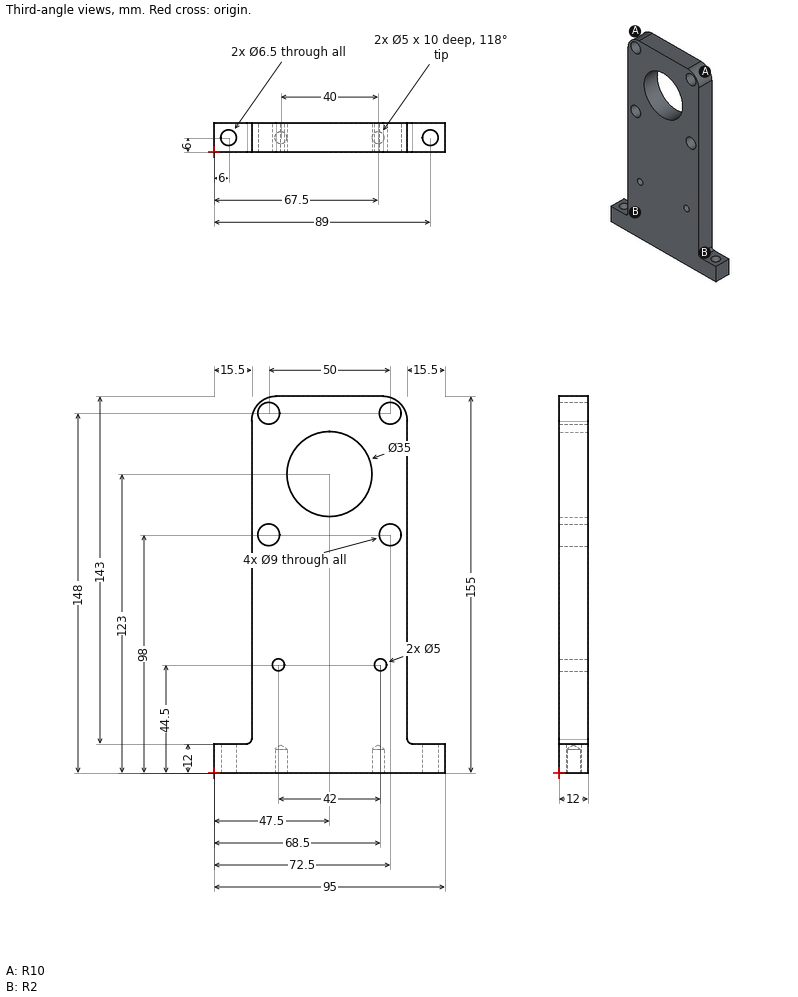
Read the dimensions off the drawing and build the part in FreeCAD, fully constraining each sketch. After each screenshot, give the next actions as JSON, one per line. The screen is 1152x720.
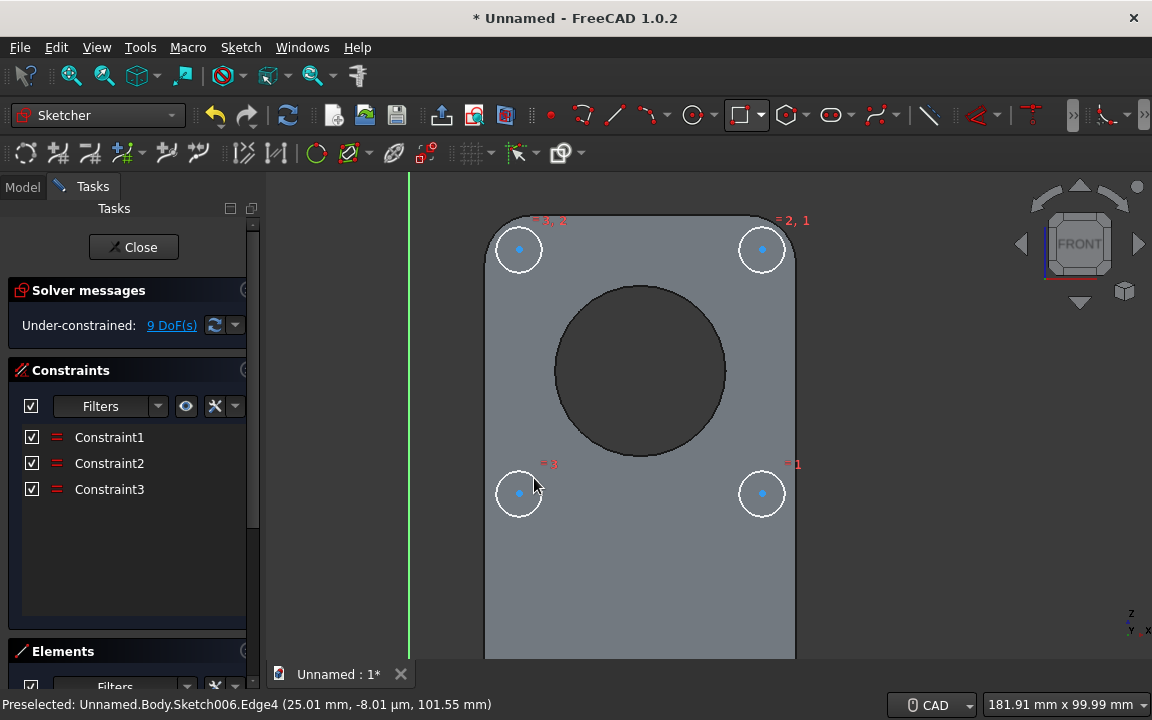
{"action": "left_click", "coordinate": [762, 494]}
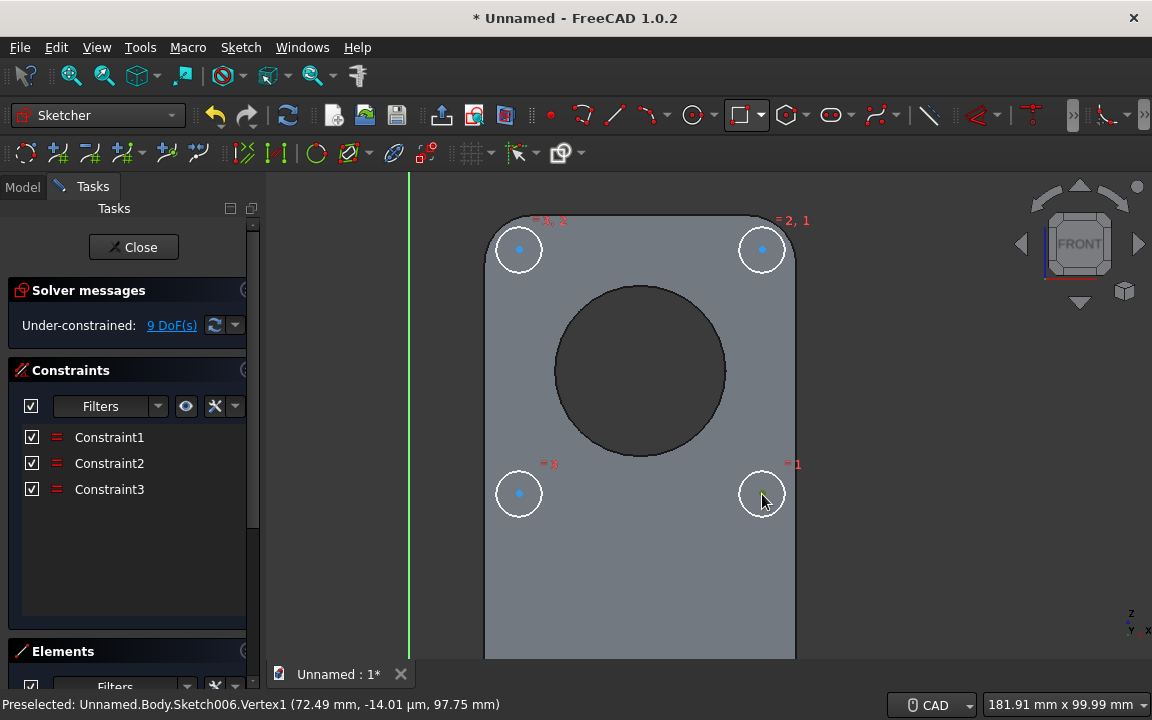
{"action": "left_click", "coordinate": [762, 250]}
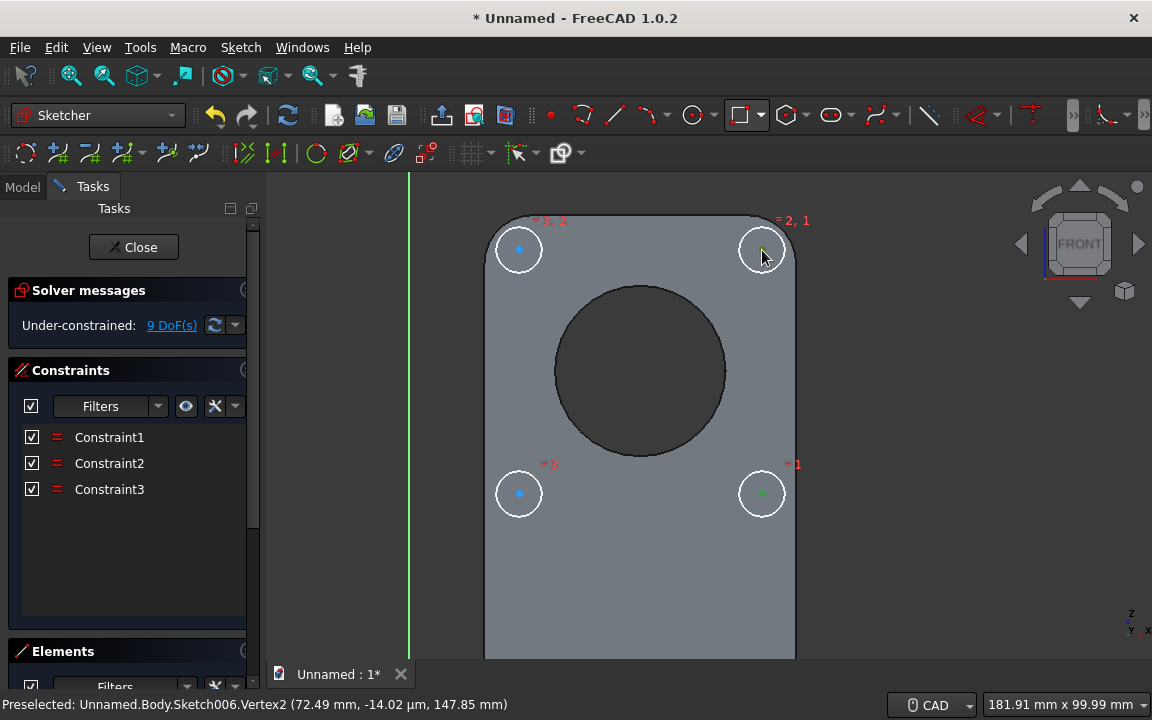
{"action": "key", "text": "v"}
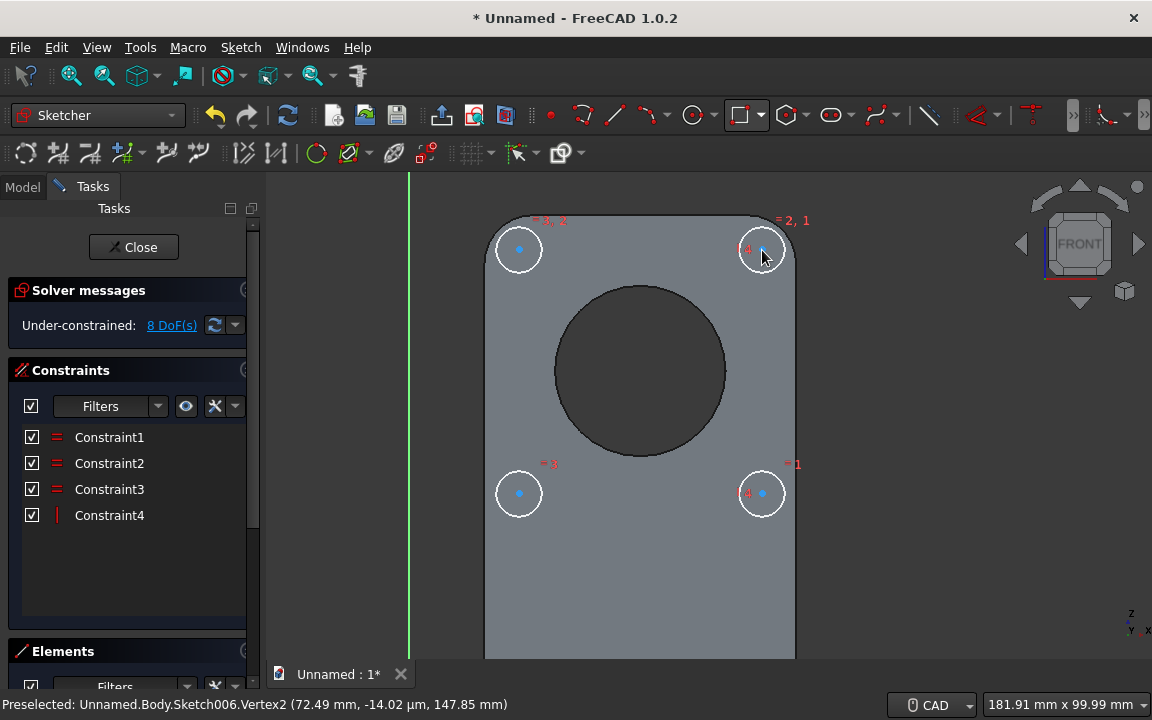
{"action": "left_click", "coordinate": [762, 250]}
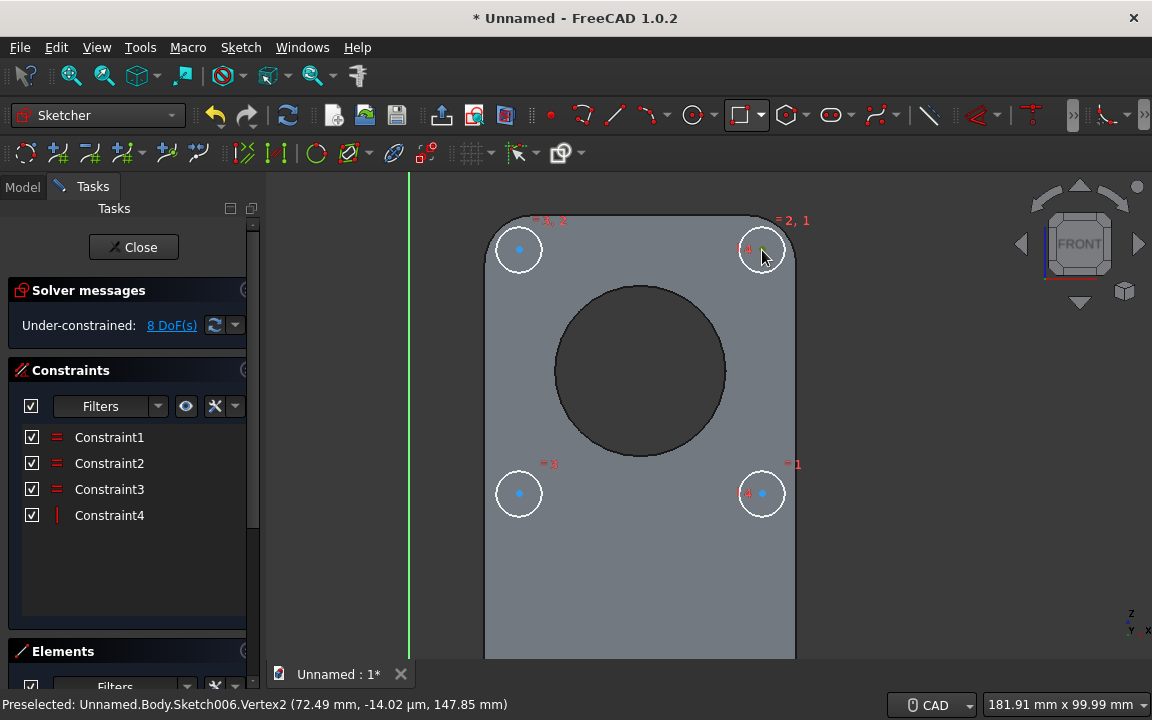
{"action": "left_click", "coordinate": [519, 250]}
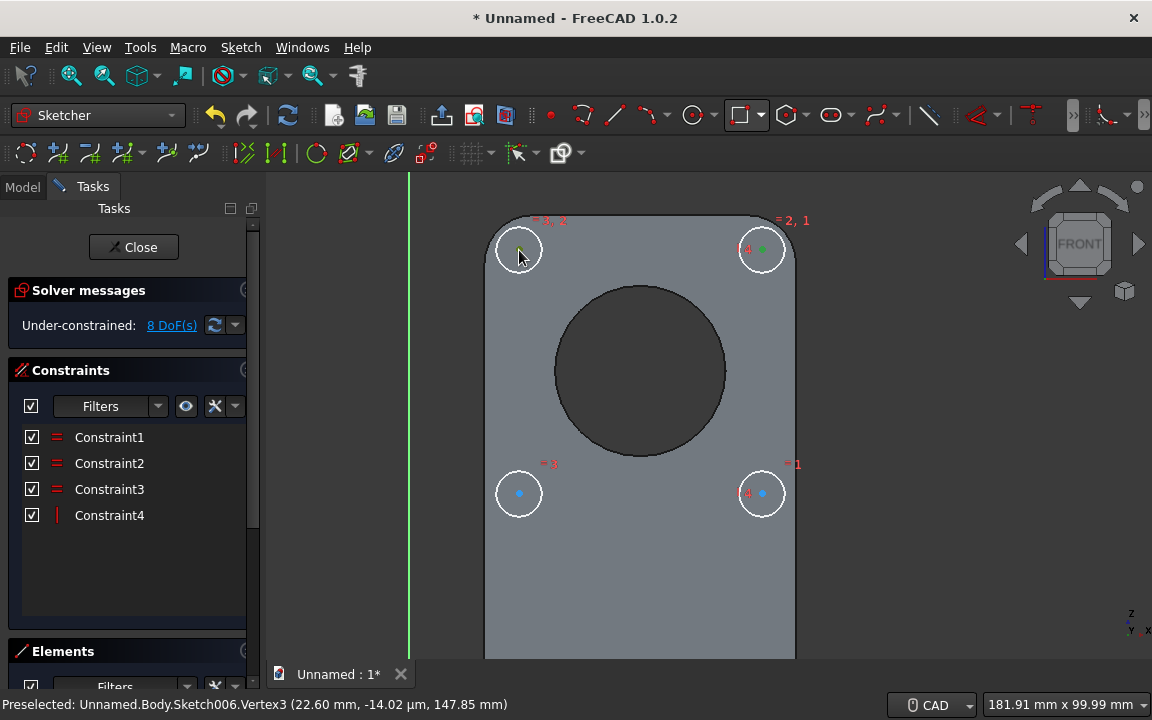
{"action": "key", "text": "h"}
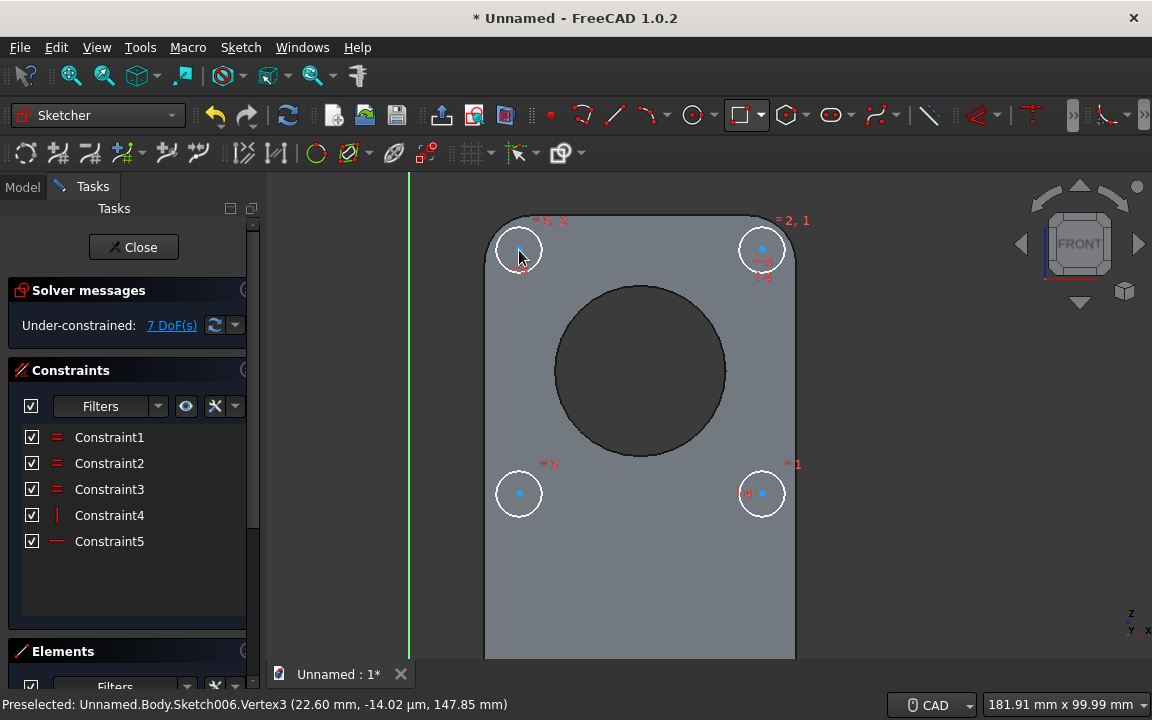
{"action": "left_click", "coordinate": [519, 250]}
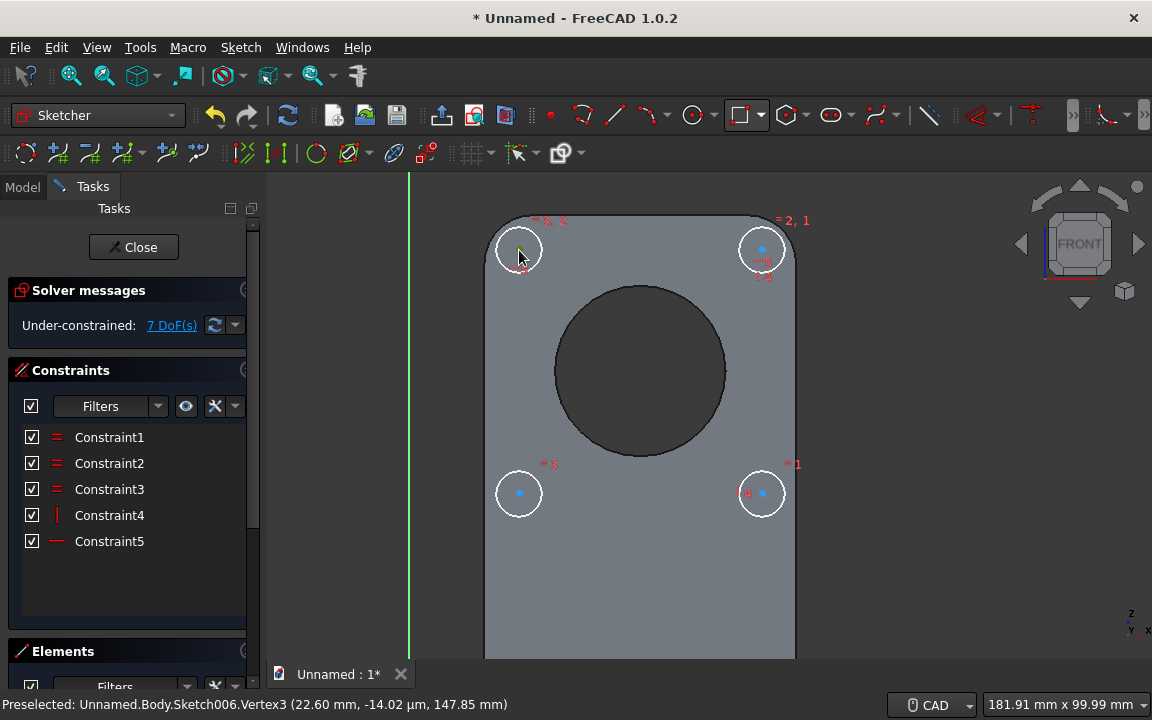
{"action": "left_click", "coordinate": [519, 494]}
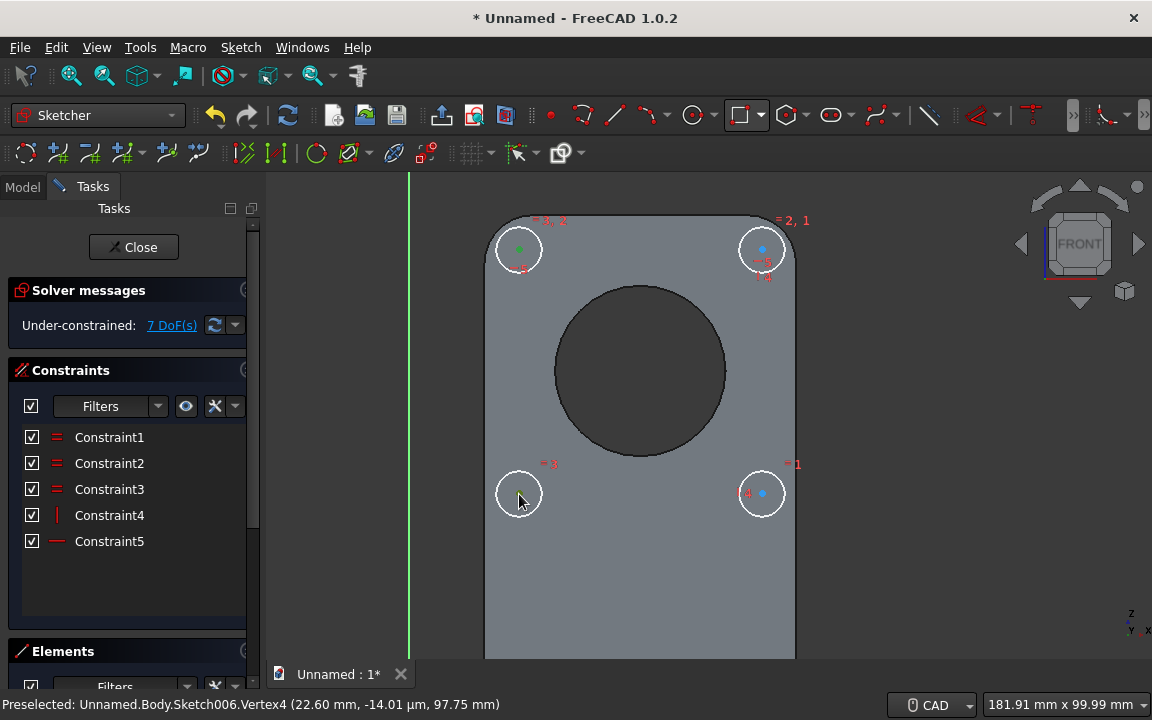
{"action": "key", "text": "v"}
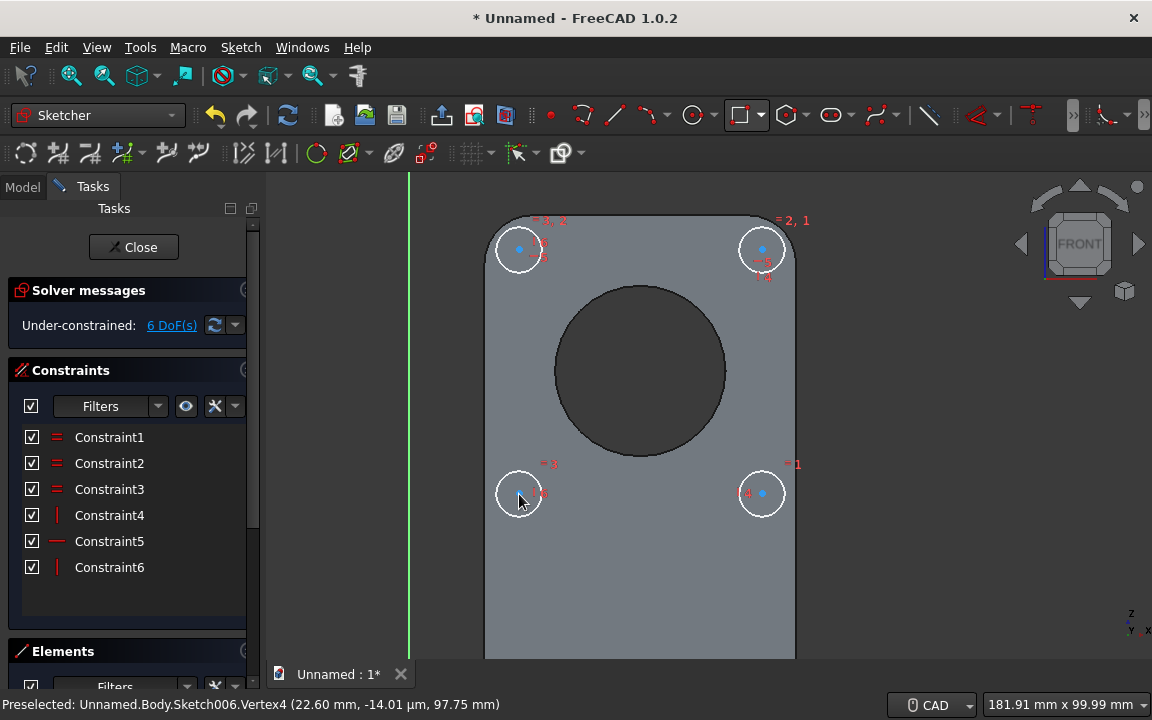
{"action": "left_click", "coordinate": [762, 494]}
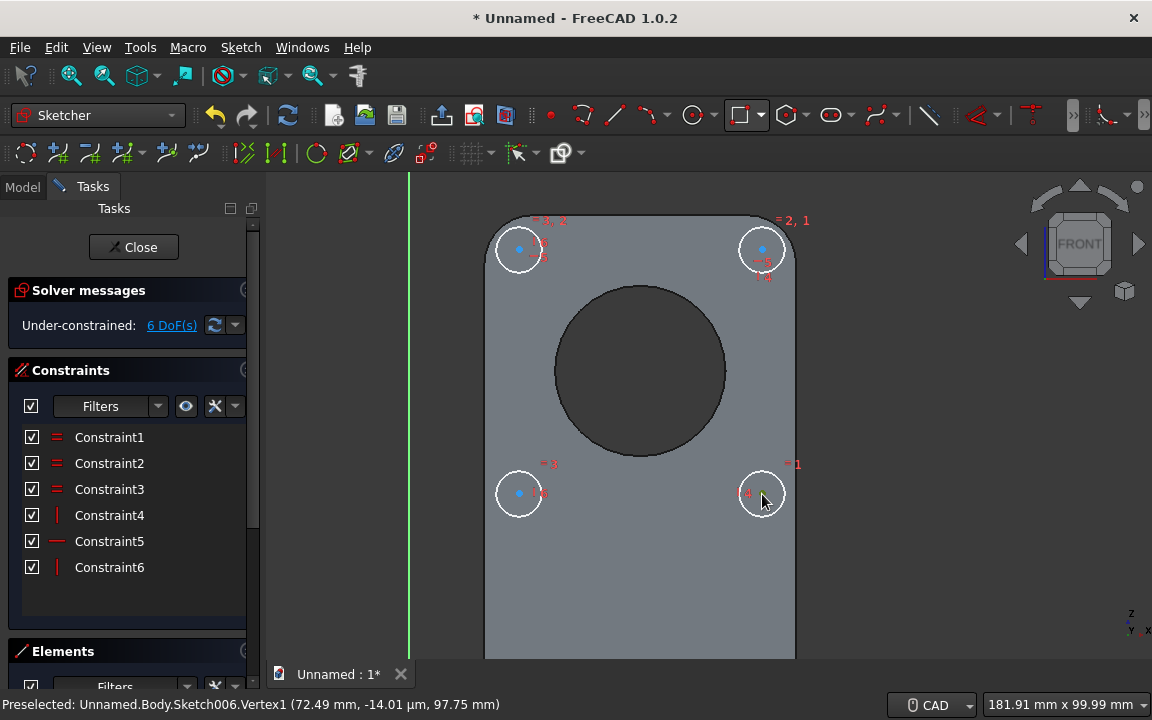
{"action": "left_click", "coordinate": [519, 494]}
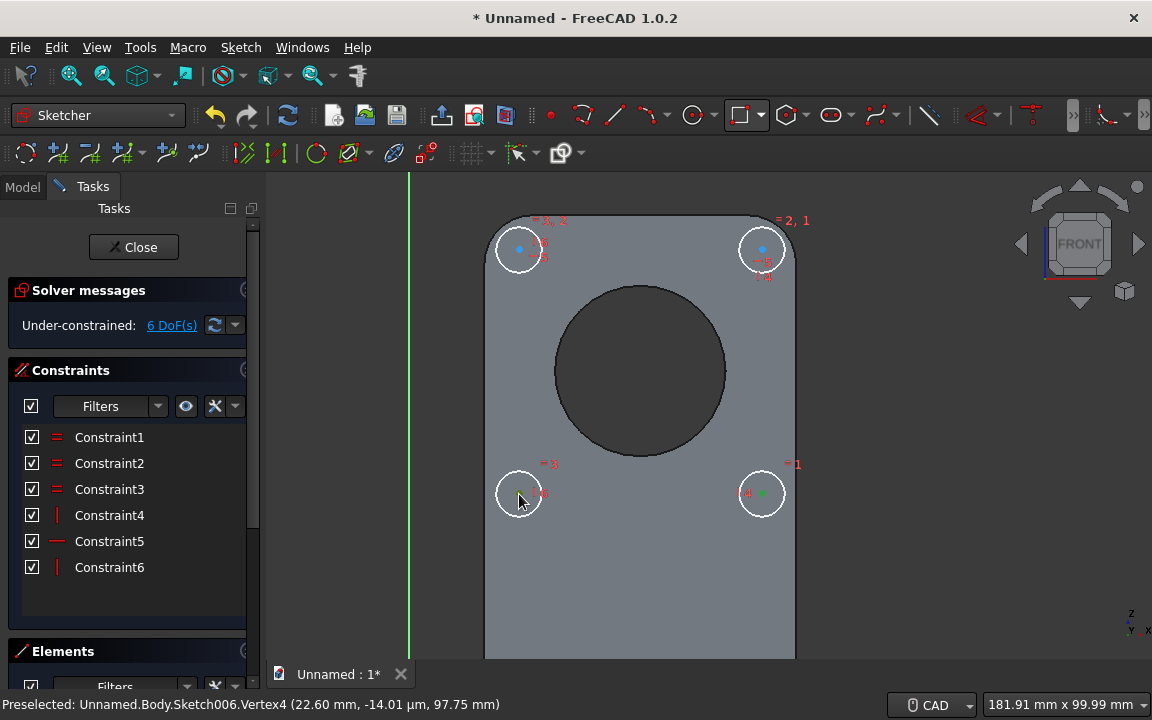
{"action": "key", "text": "h"}